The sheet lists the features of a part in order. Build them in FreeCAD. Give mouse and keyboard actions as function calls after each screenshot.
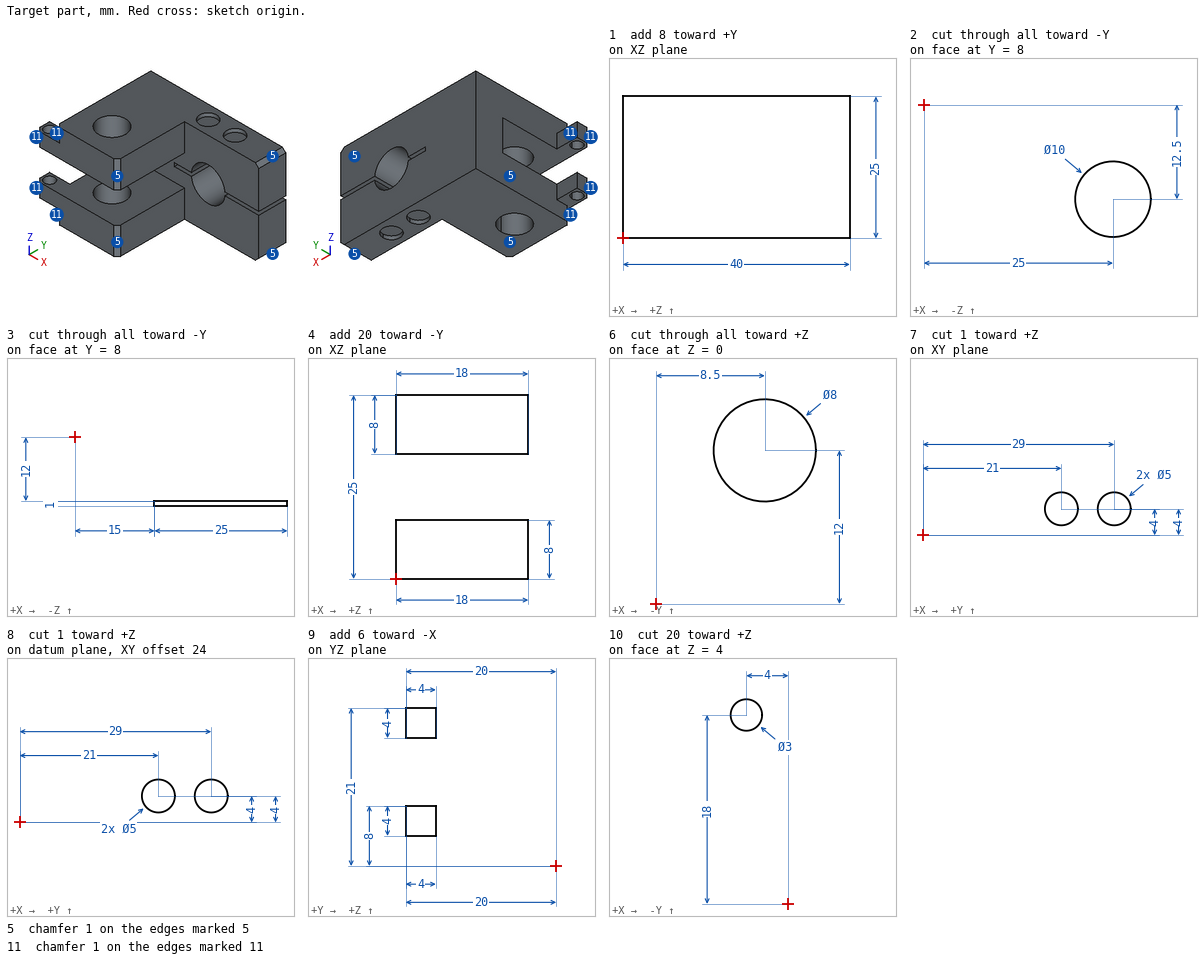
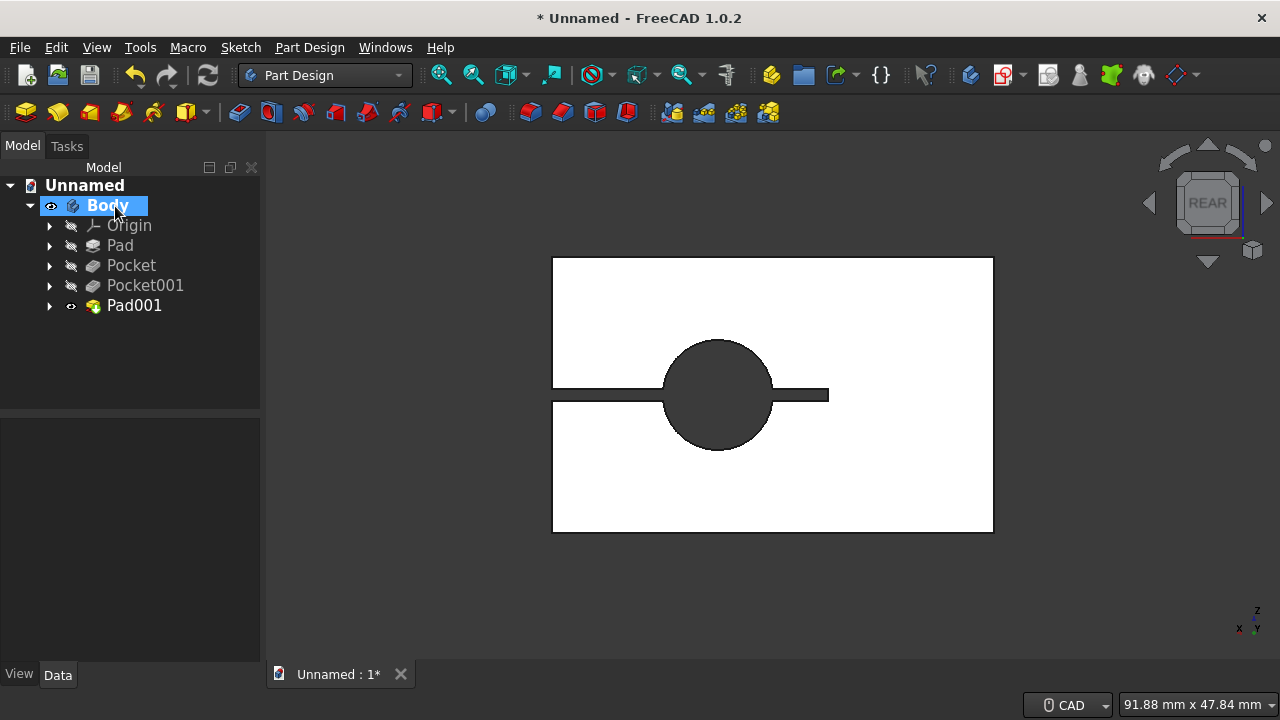
key(0)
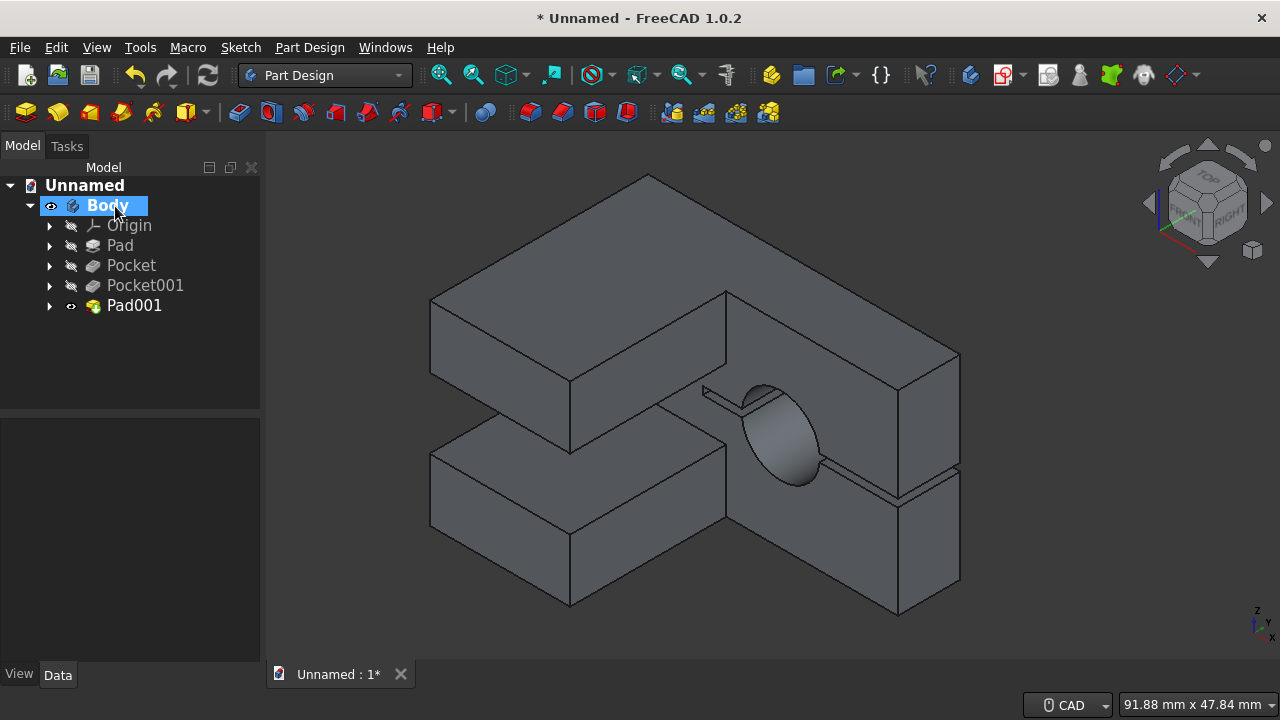
click(442, 76)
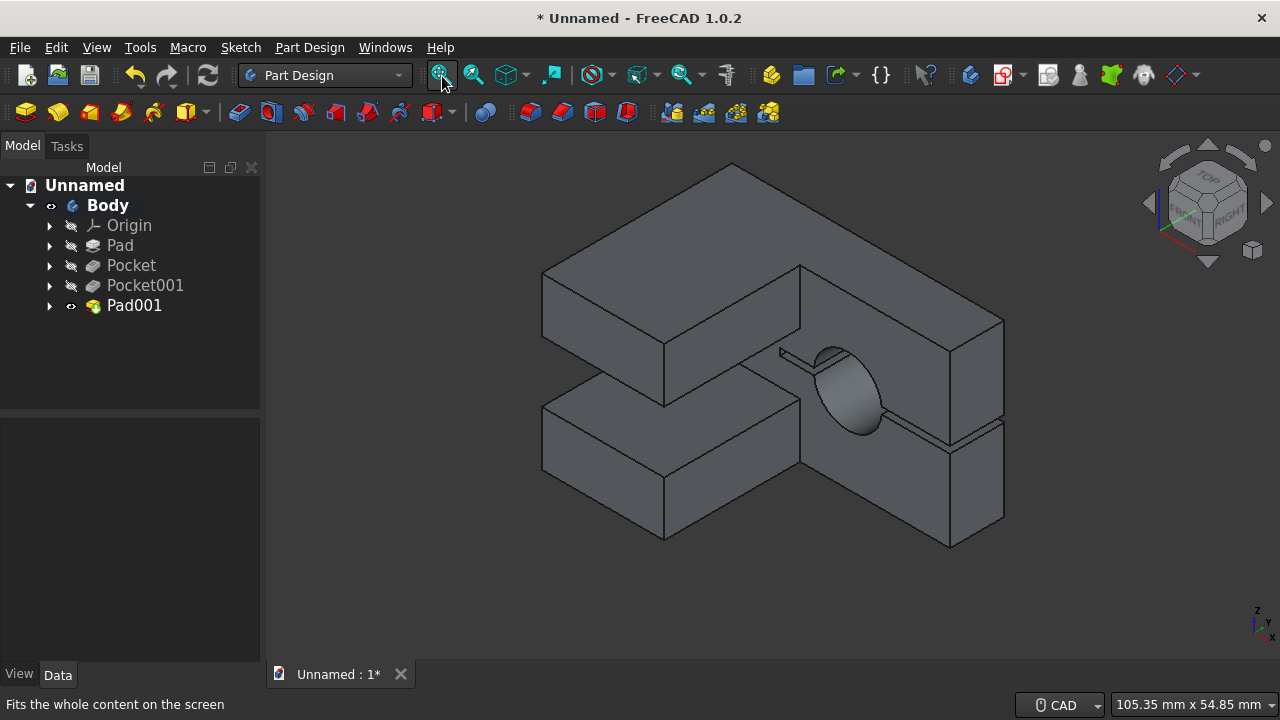
click(664, 508)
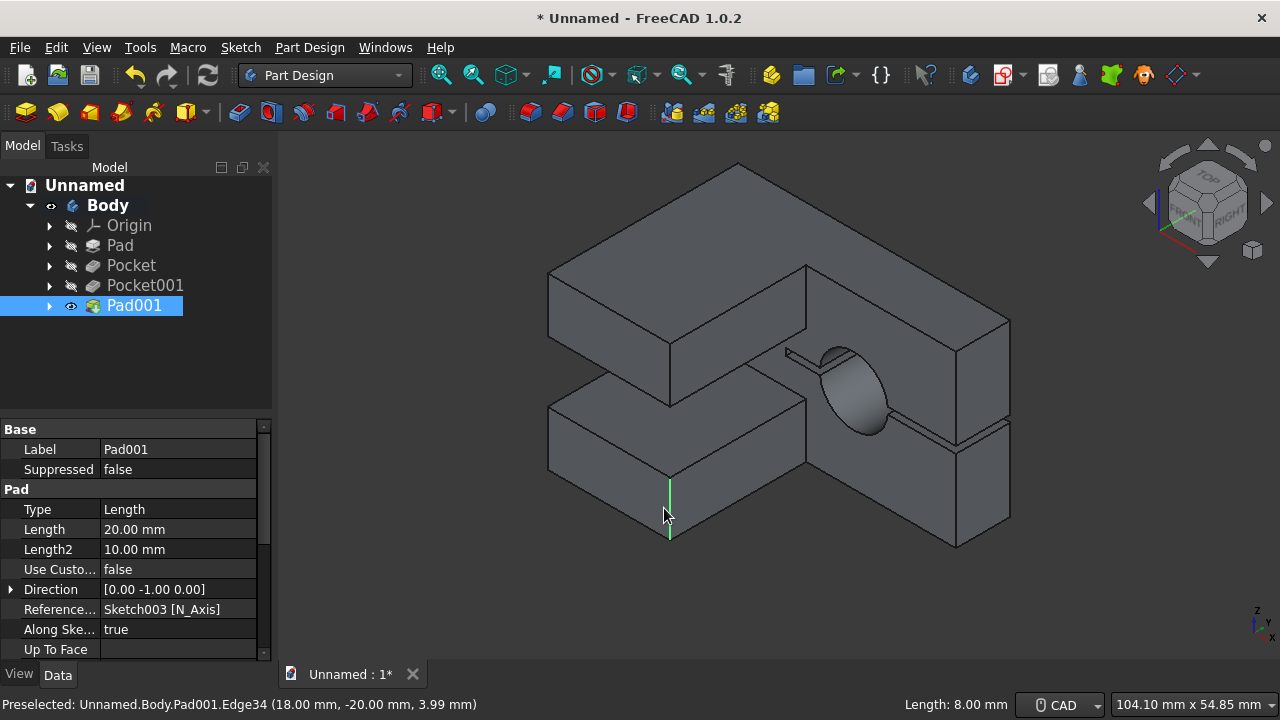
click(670, 374, ctrl)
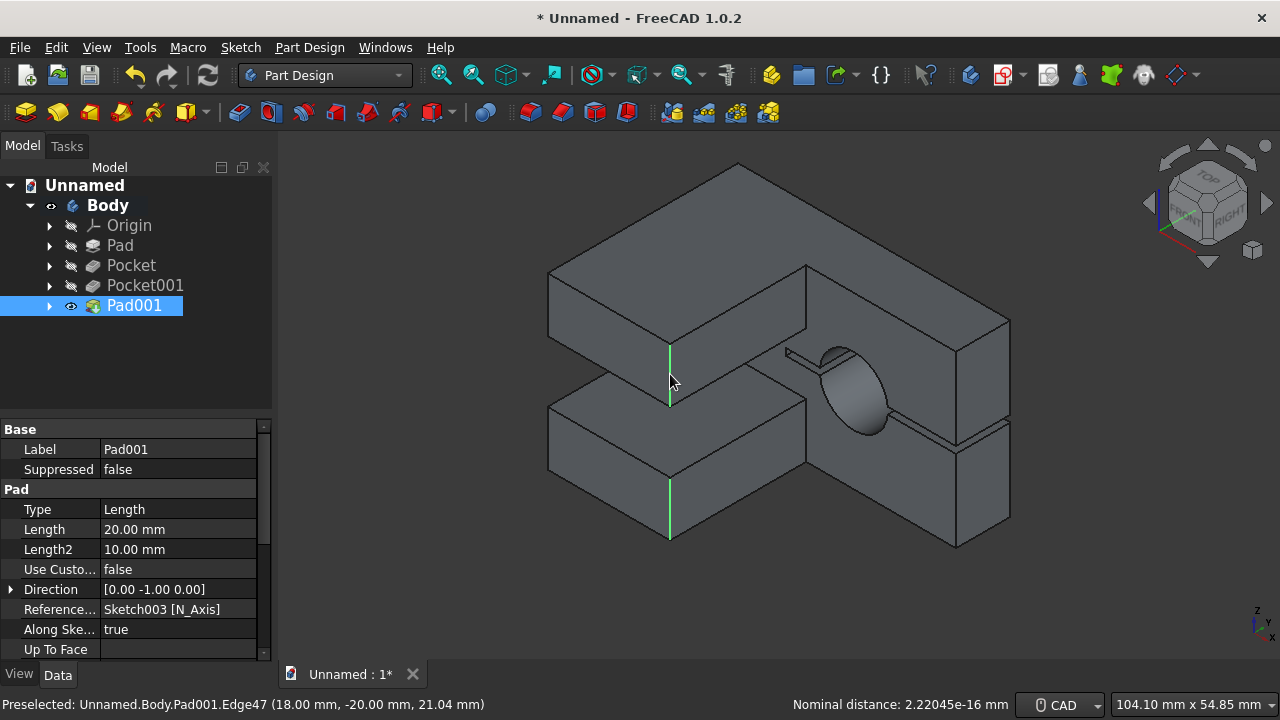
click(983, 335, ctrl)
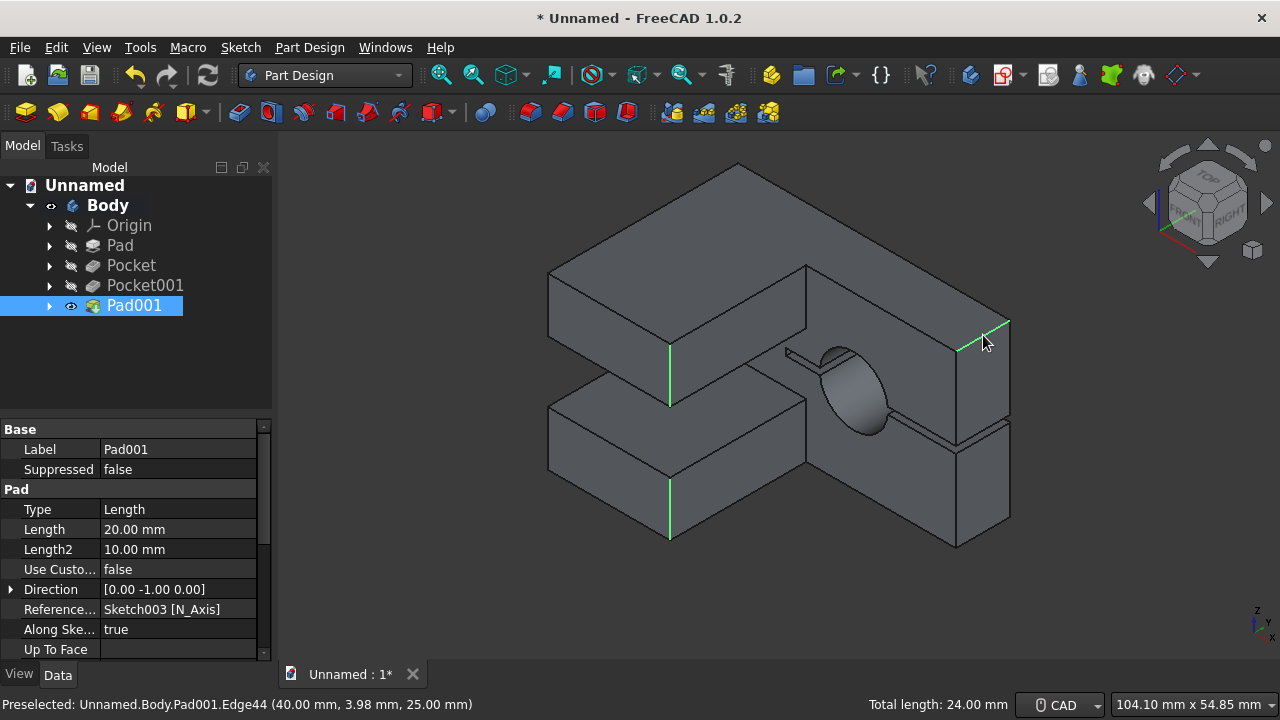
key(2)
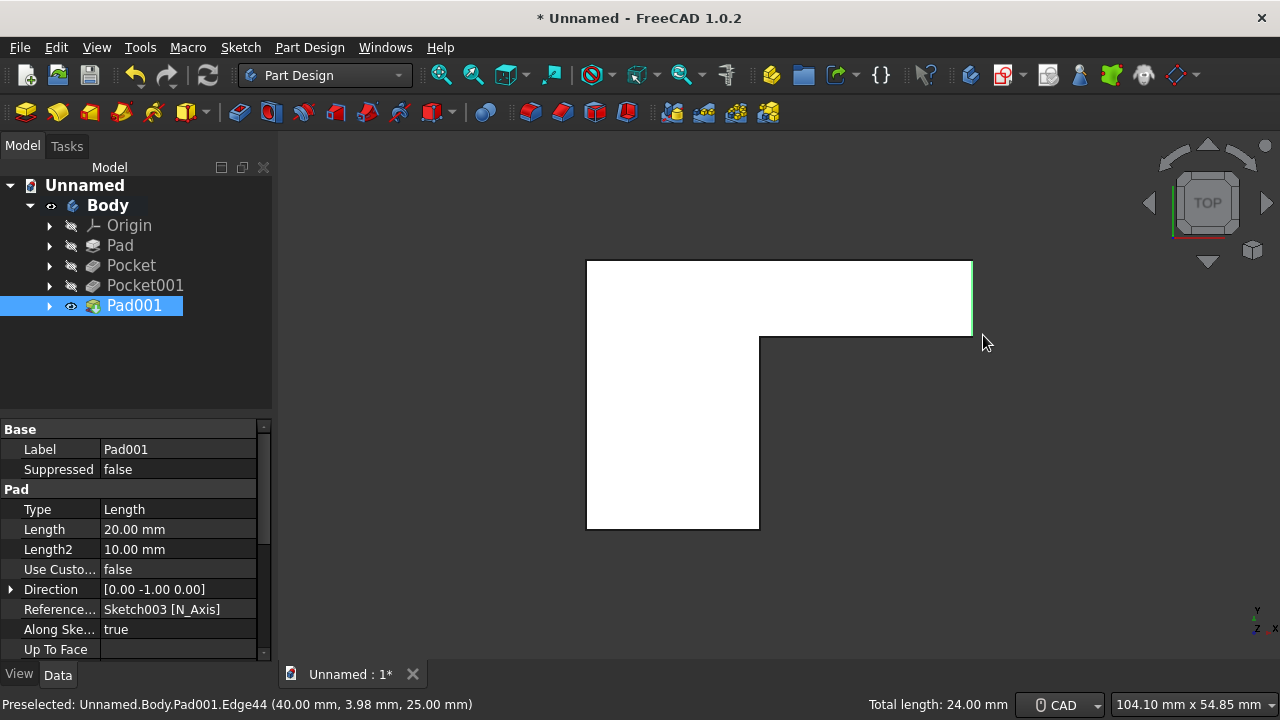
key(1)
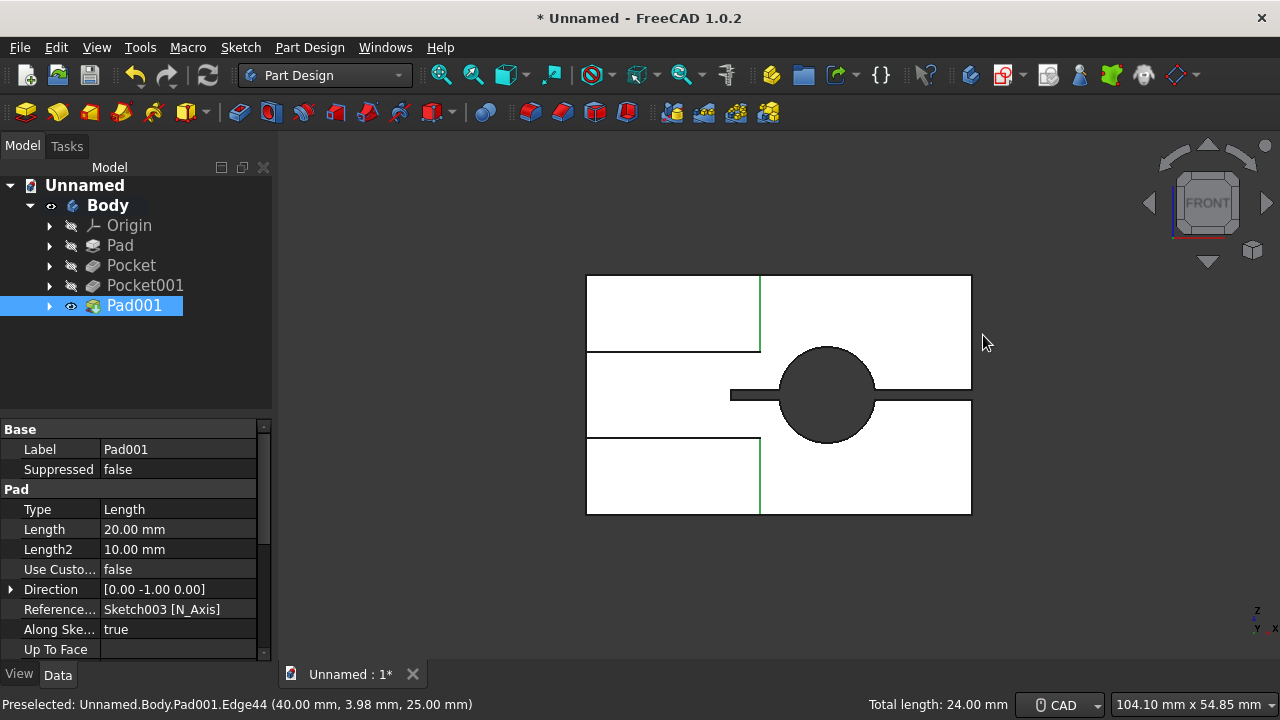
key(3)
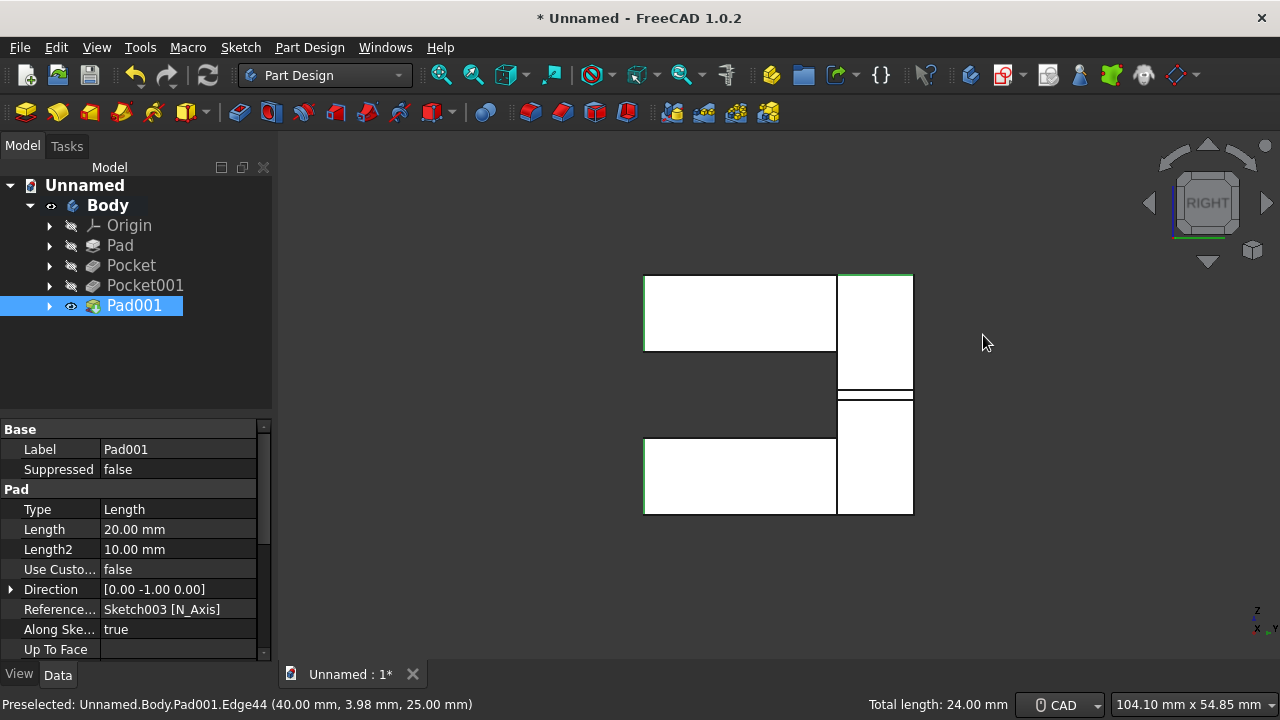
click(875, 514, ctrl)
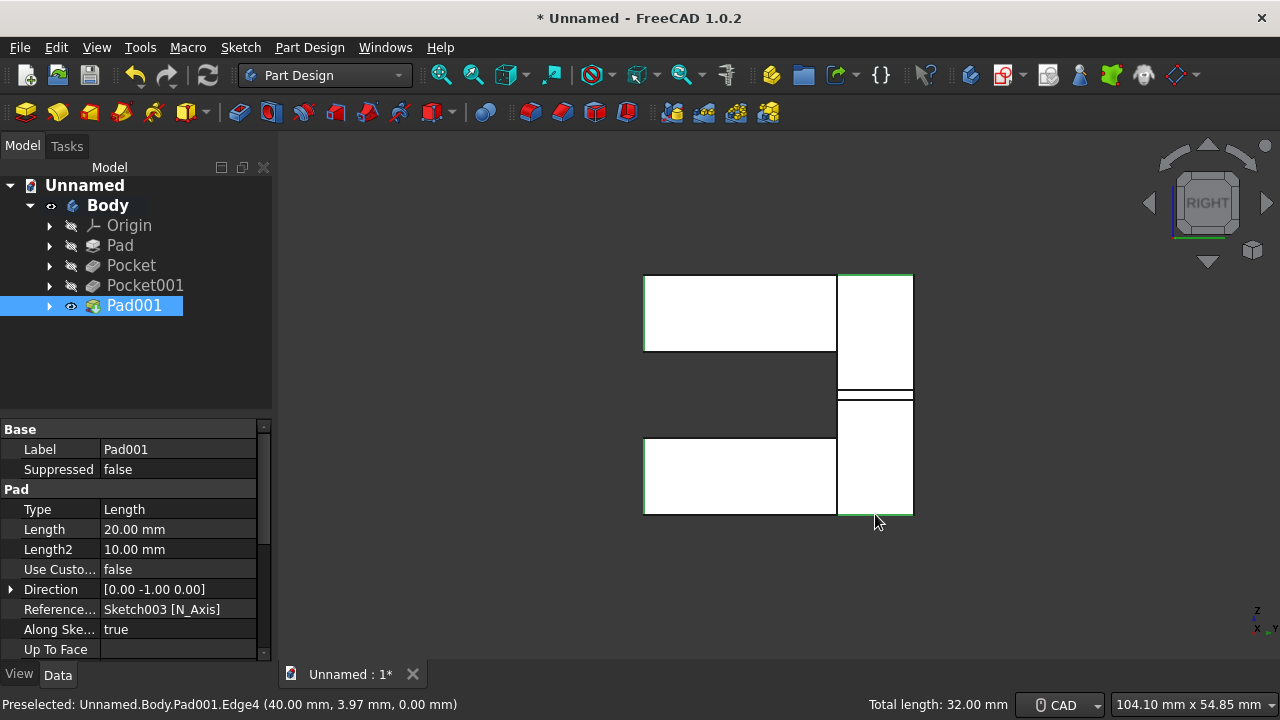
click(564, 112)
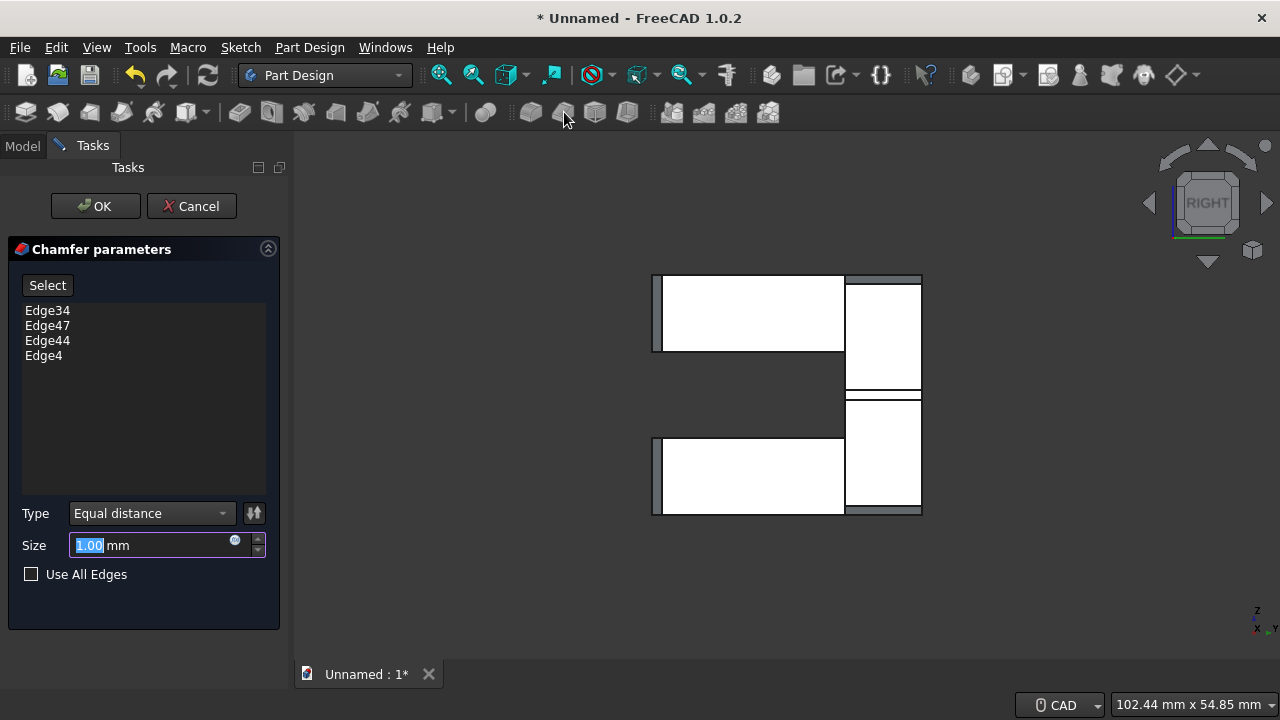
text(1)
key(Tab)